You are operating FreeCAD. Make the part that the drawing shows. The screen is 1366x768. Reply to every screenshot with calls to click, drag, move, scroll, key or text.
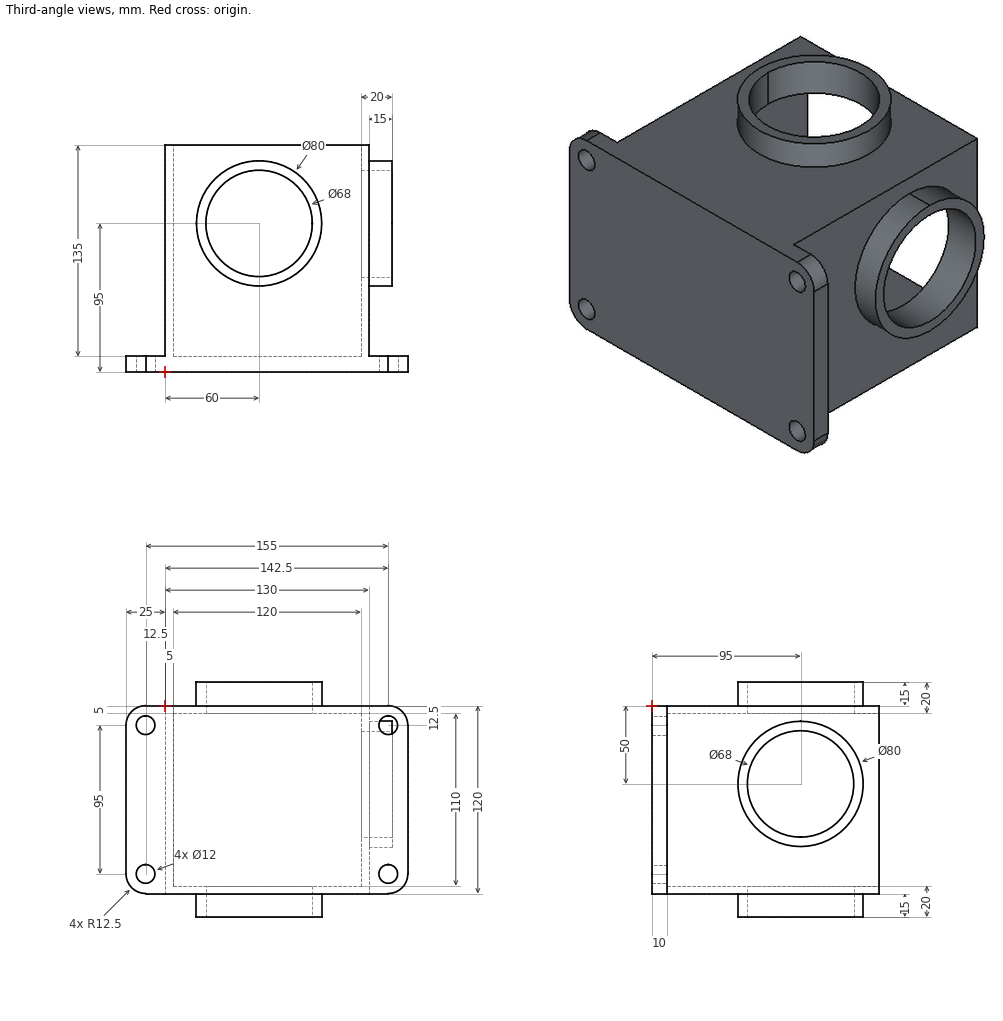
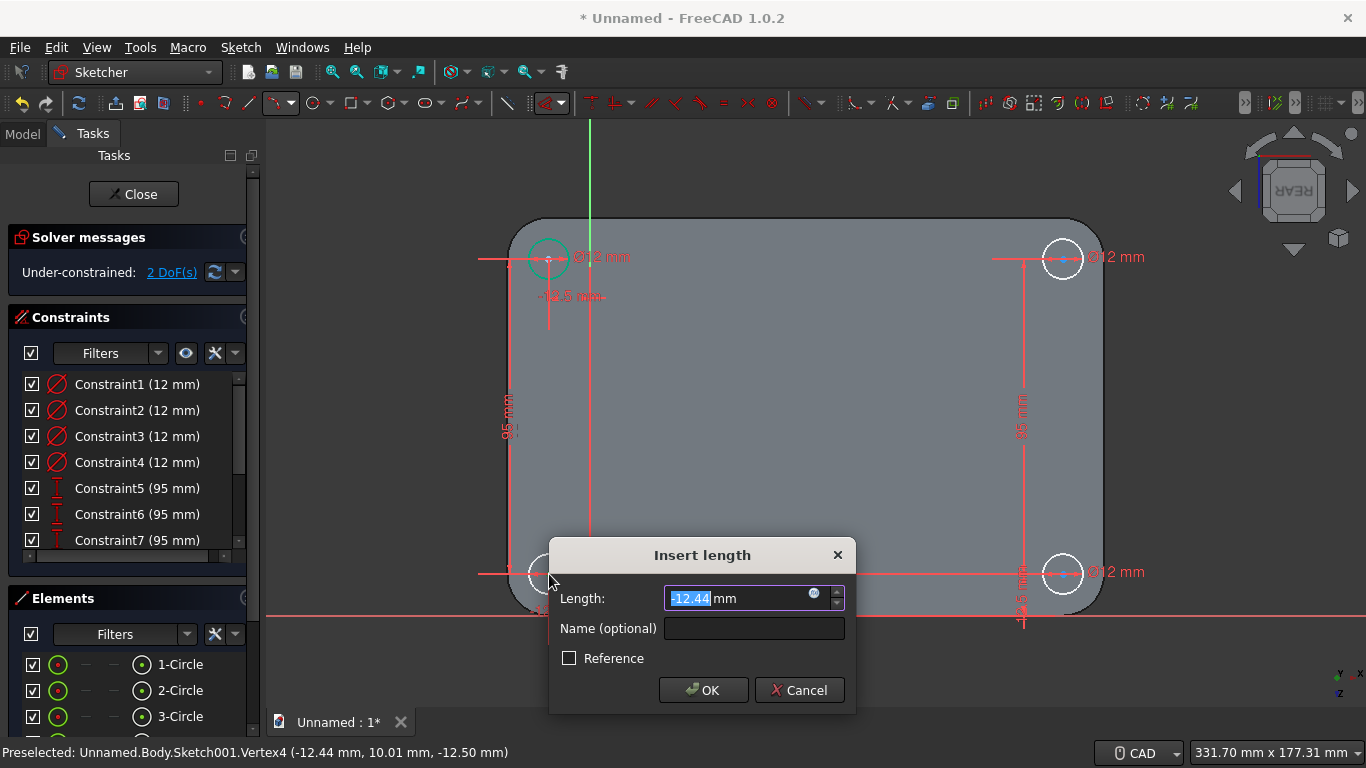
text(-12.5)
key(Return)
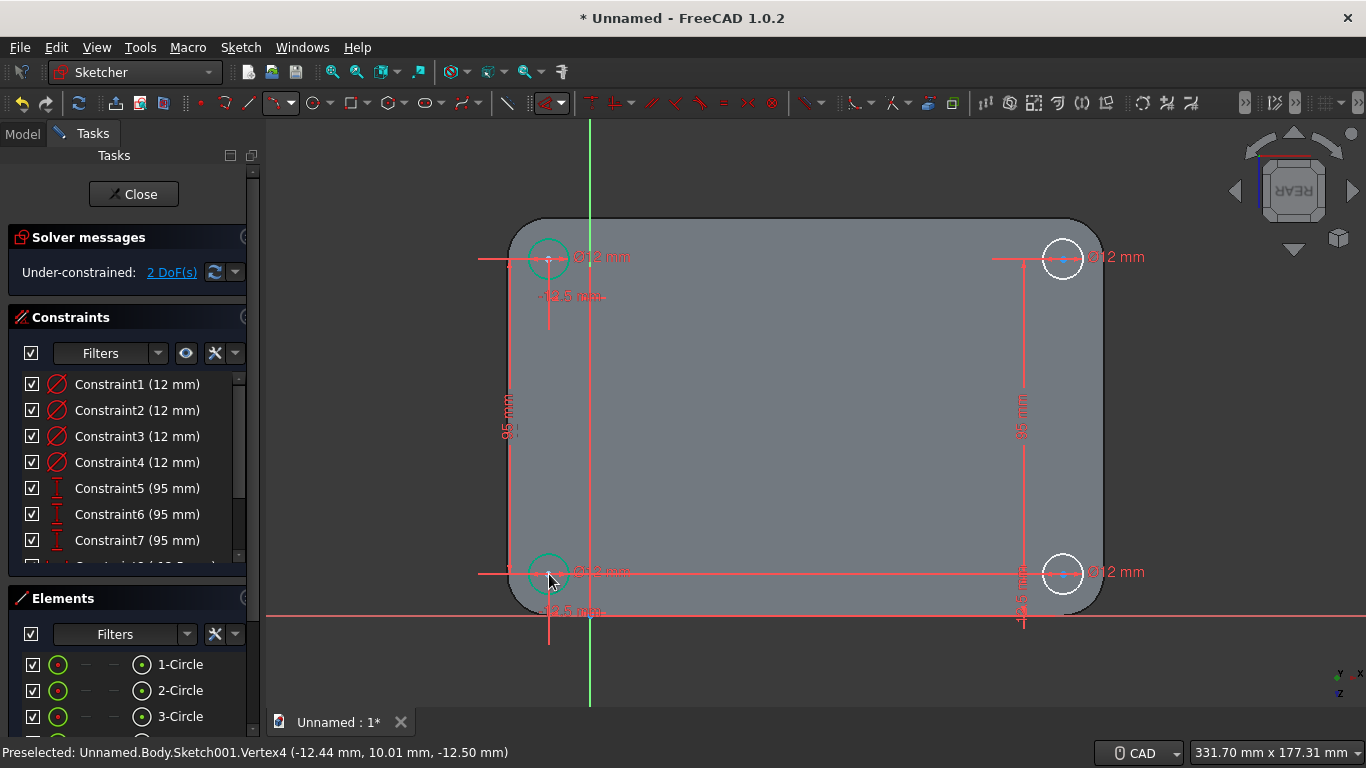
click(549, 259)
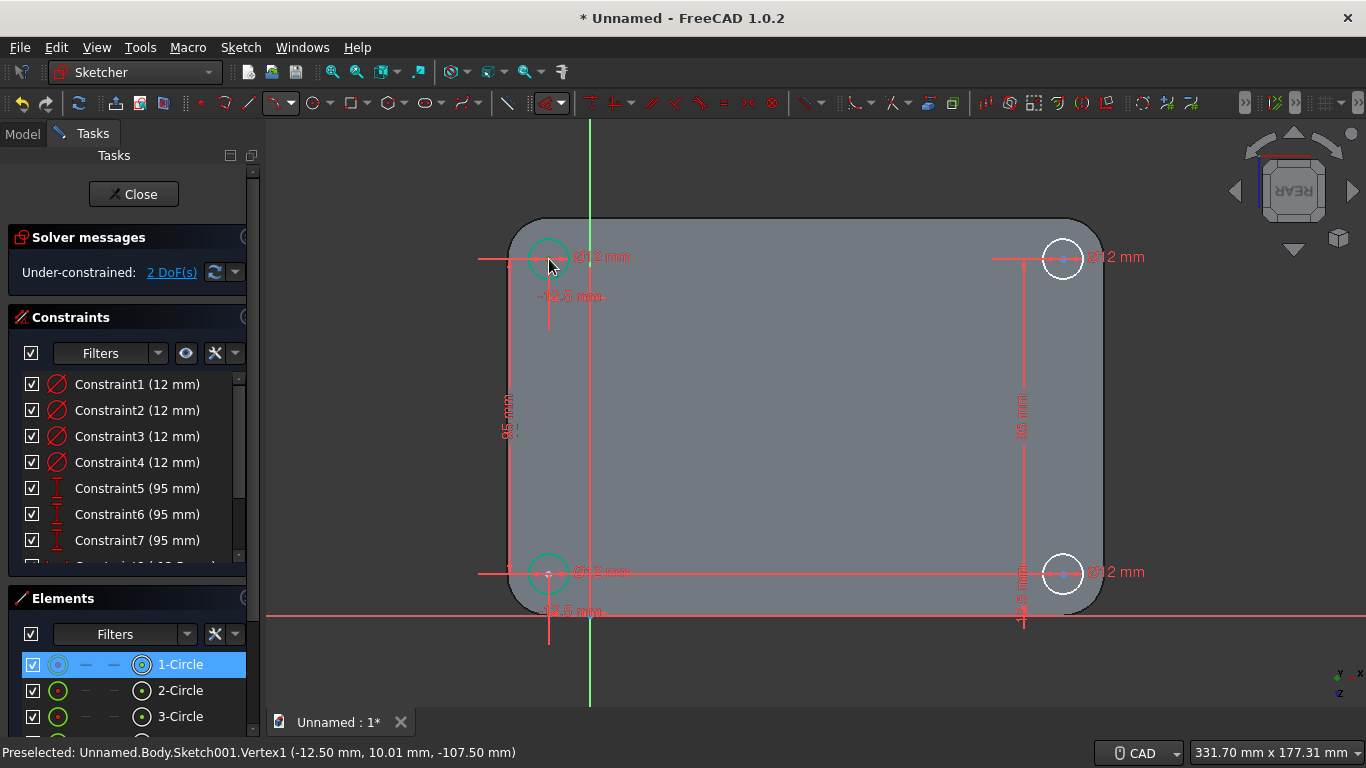
click(1063, 259)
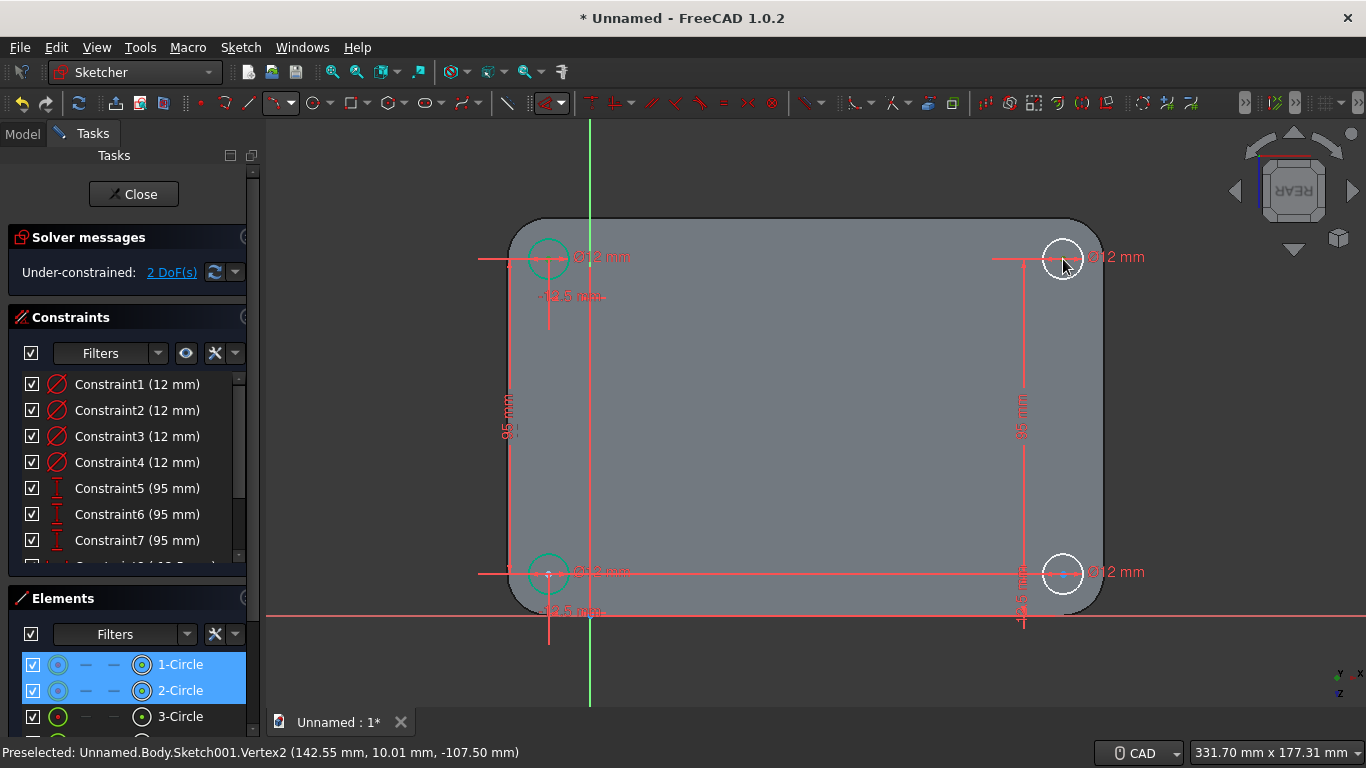
key(l)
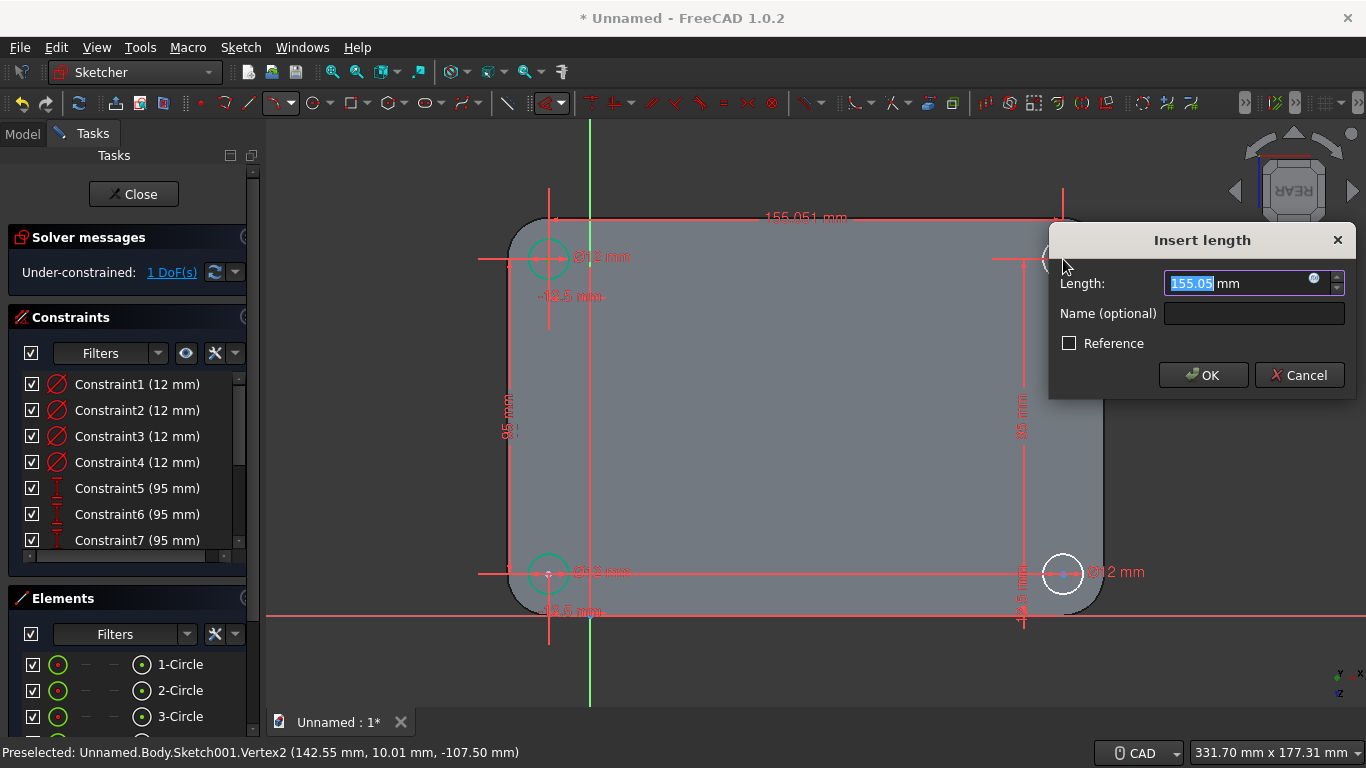
text(155)
key(Return)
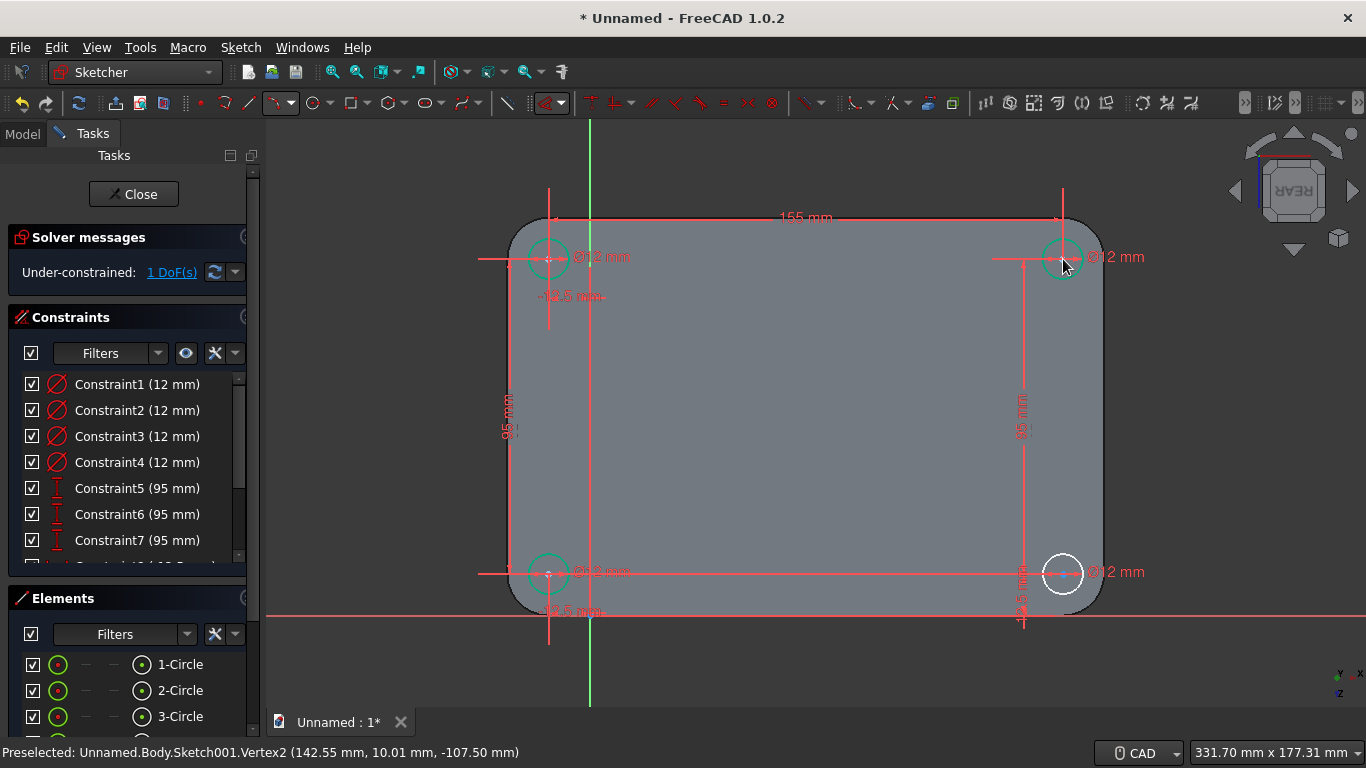
click(549, 259)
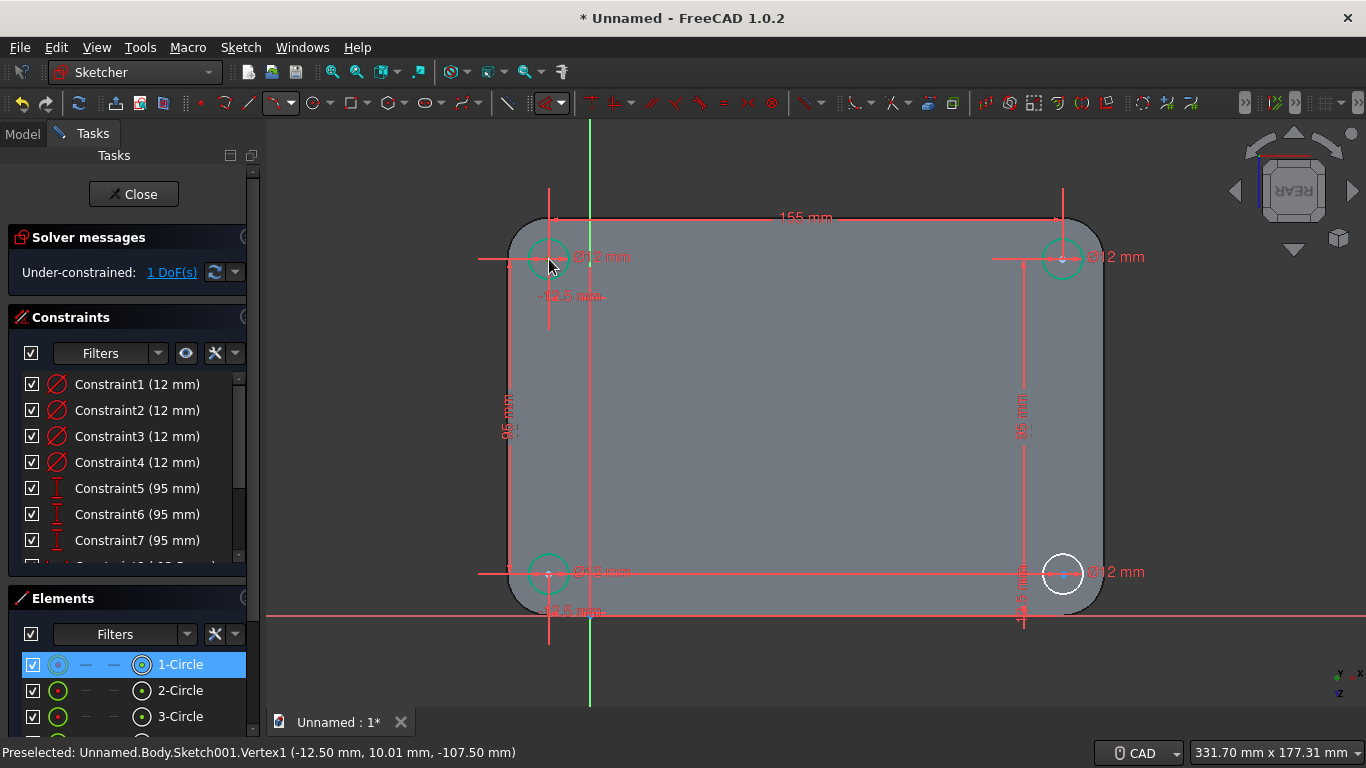
click(1063, 574)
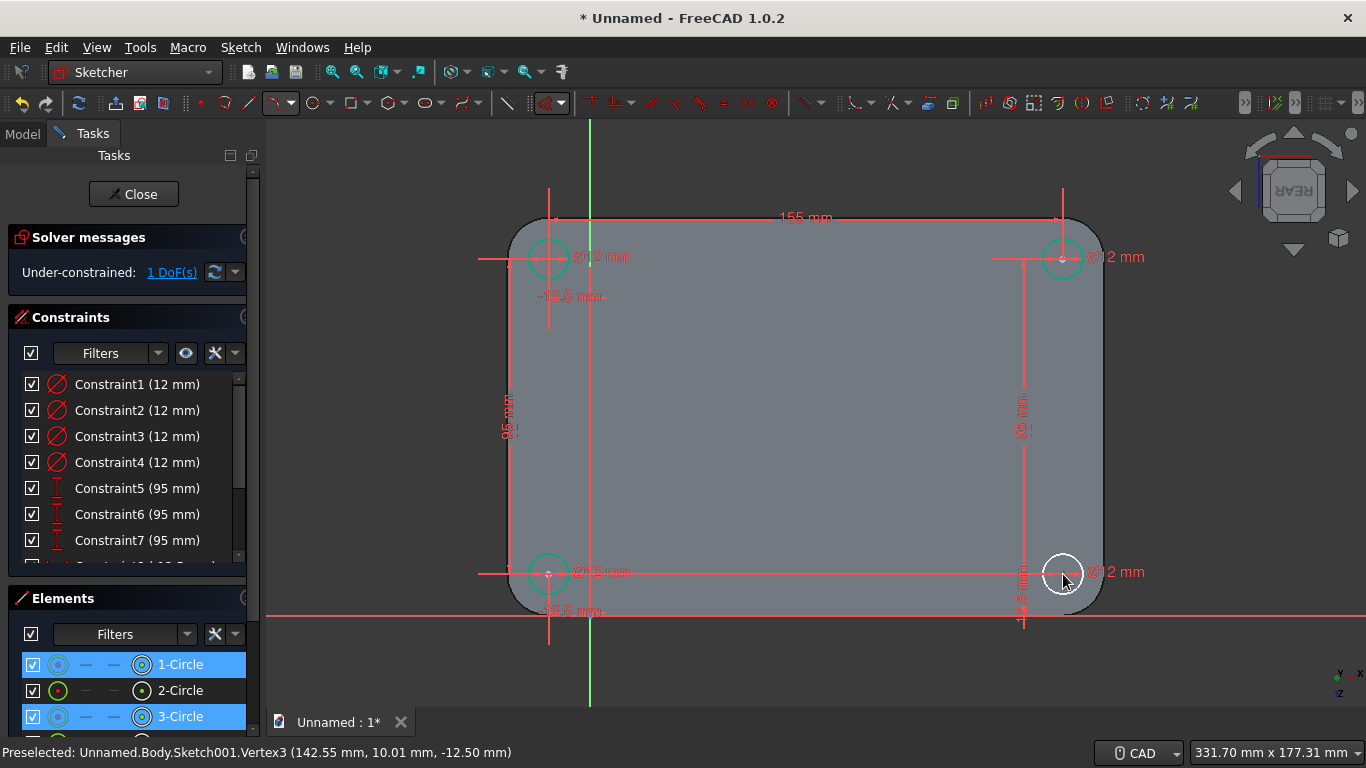
click(564, 104)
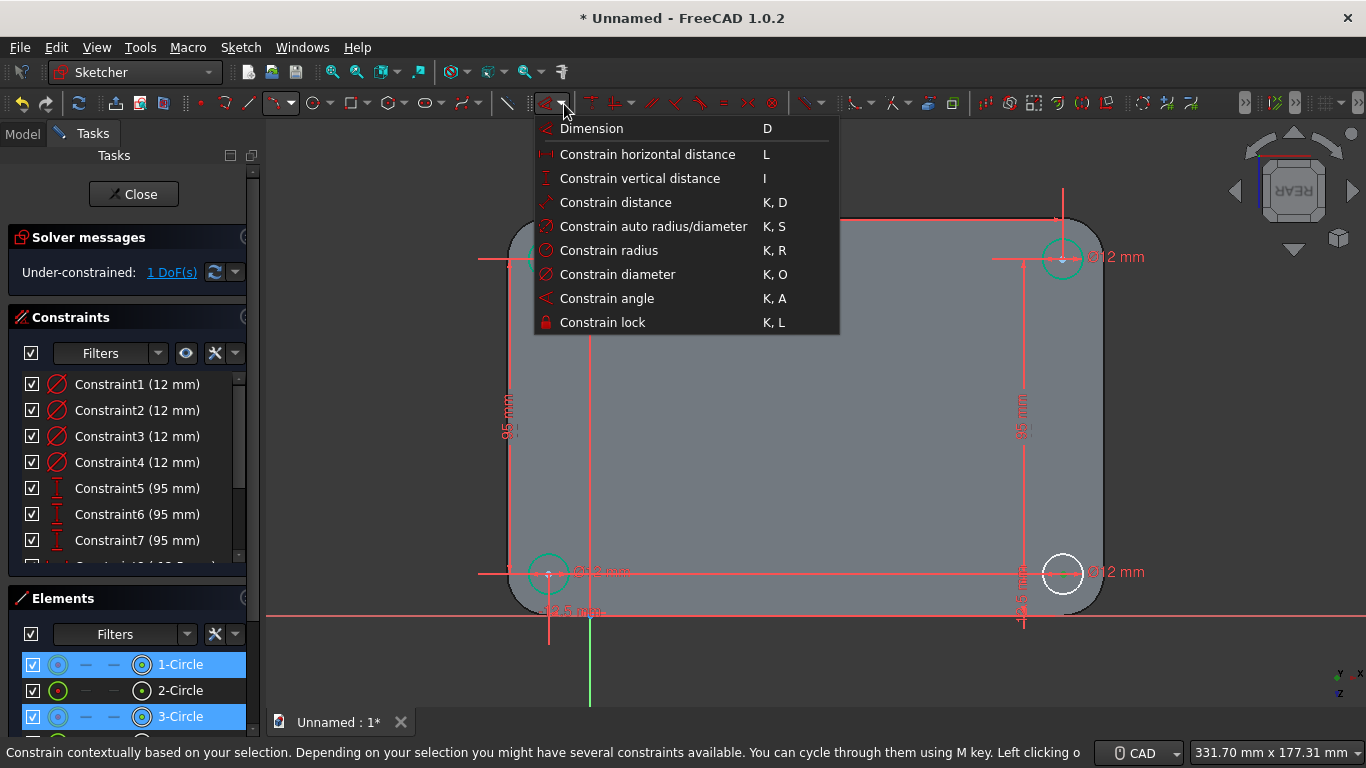
click(687, 154)